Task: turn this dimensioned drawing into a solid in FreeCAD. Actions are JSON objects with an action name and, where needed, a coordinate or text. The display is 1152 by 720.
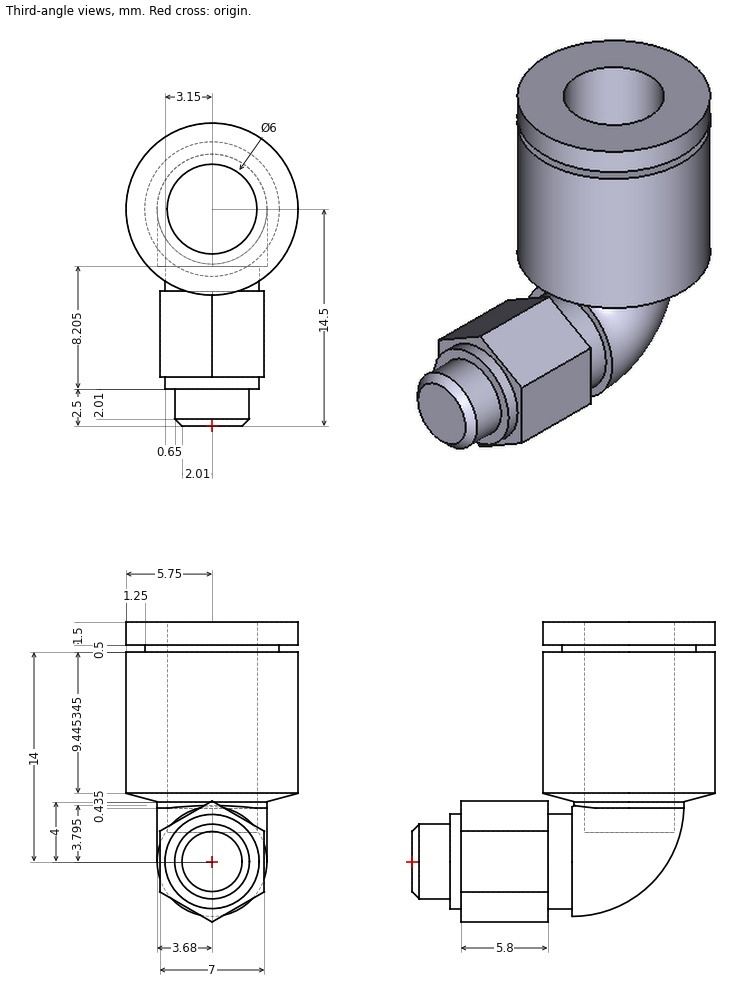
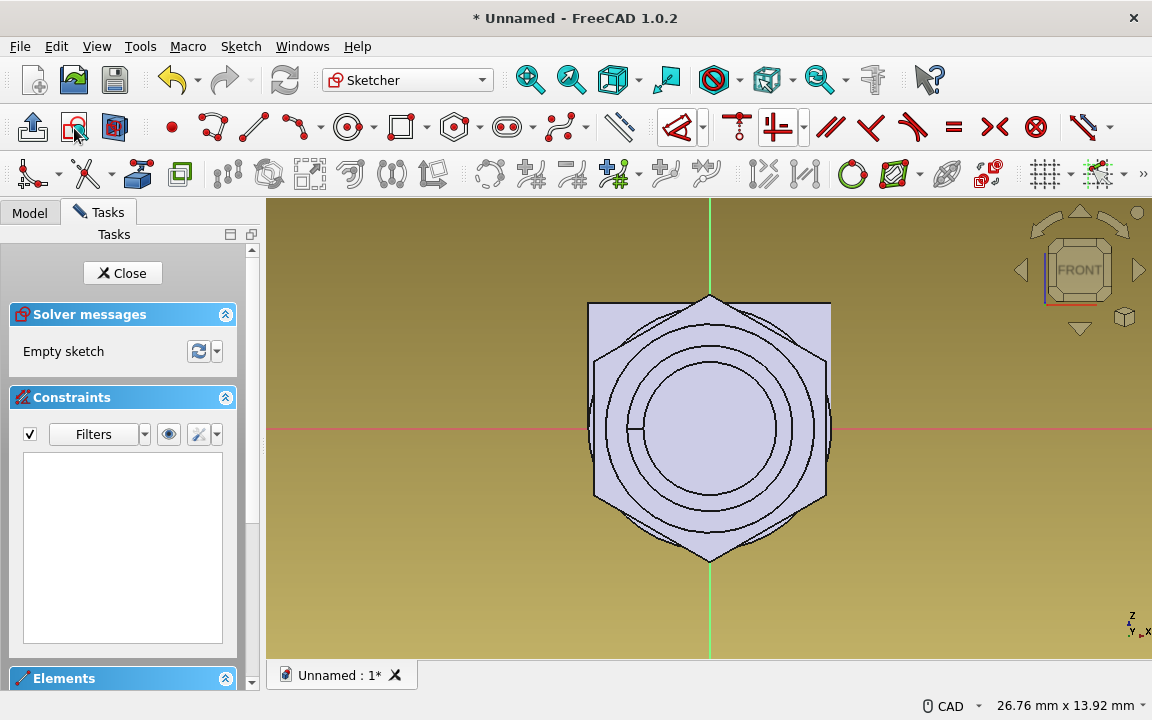
{"action": "left_click", "coordinate": [115, 128]}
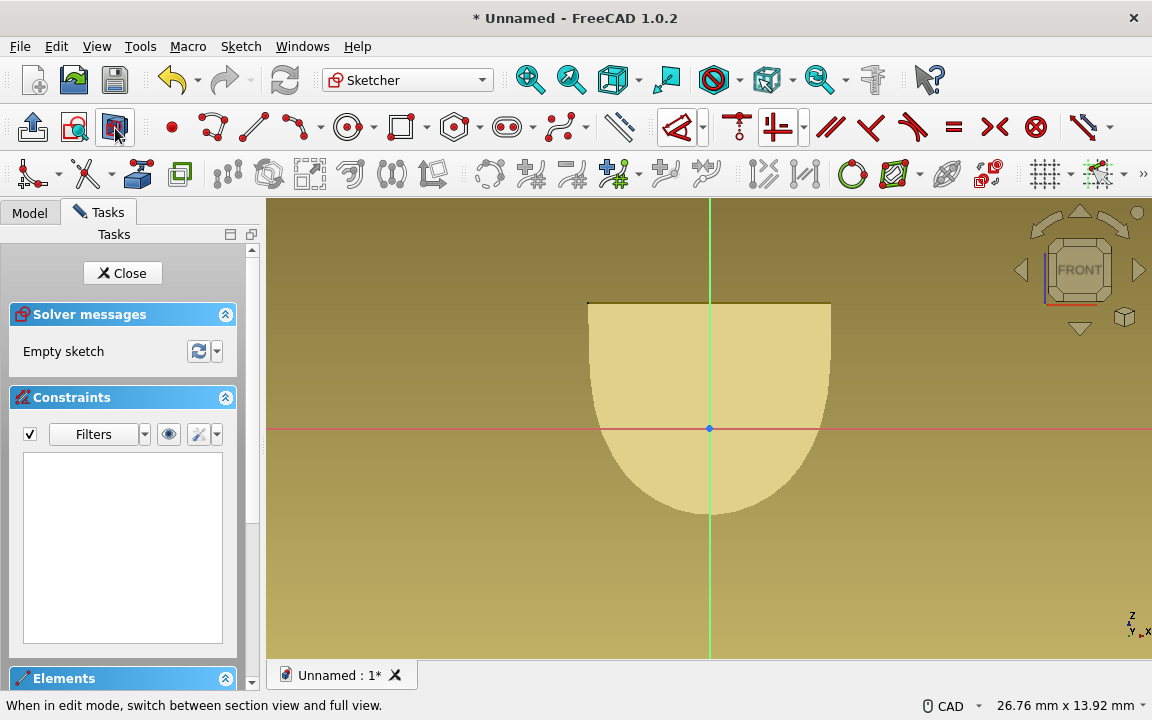
{"action": "scroll", "coordinate": [662, 631], "scroll_direction": "down", "scroll_amount": 4}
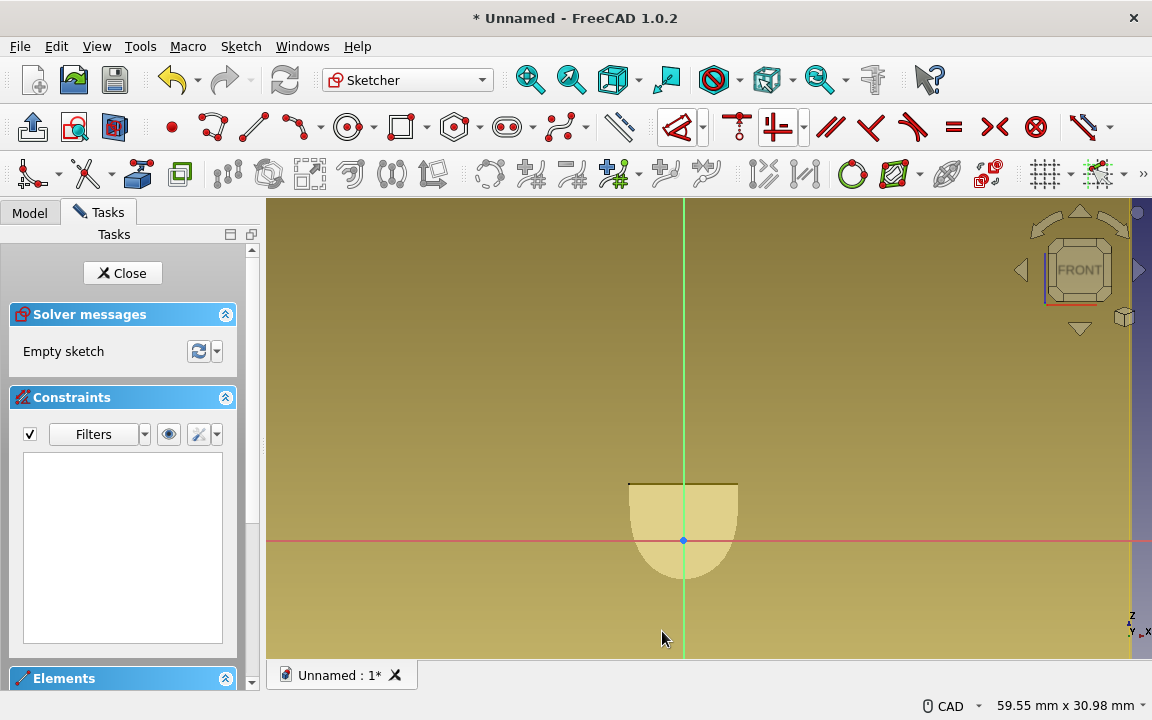
{"action": "left_click", "coordinate": [213, 128]}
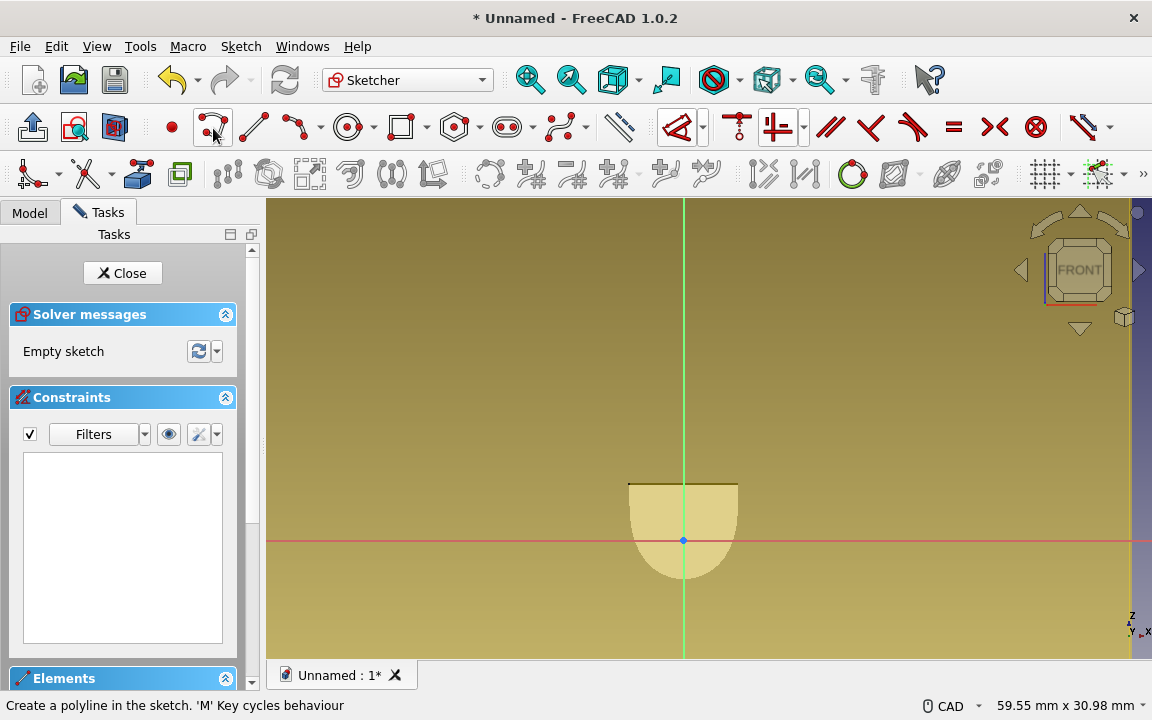
{"action": "left_click", "coordinate": [684, 487]}
{"action": "left_click", "coordinate": [629, 487]}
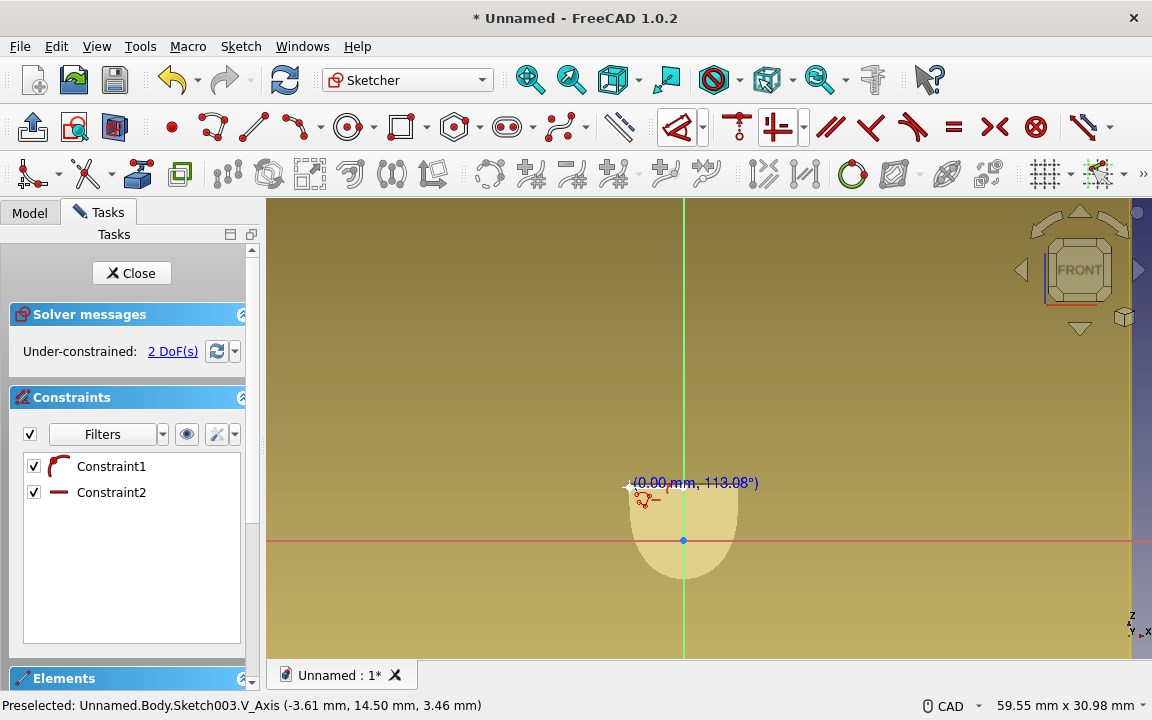
{"action": "scroll", "coordinate": [629, 481], "scroll_direction": "up", "scroll_amount": 5}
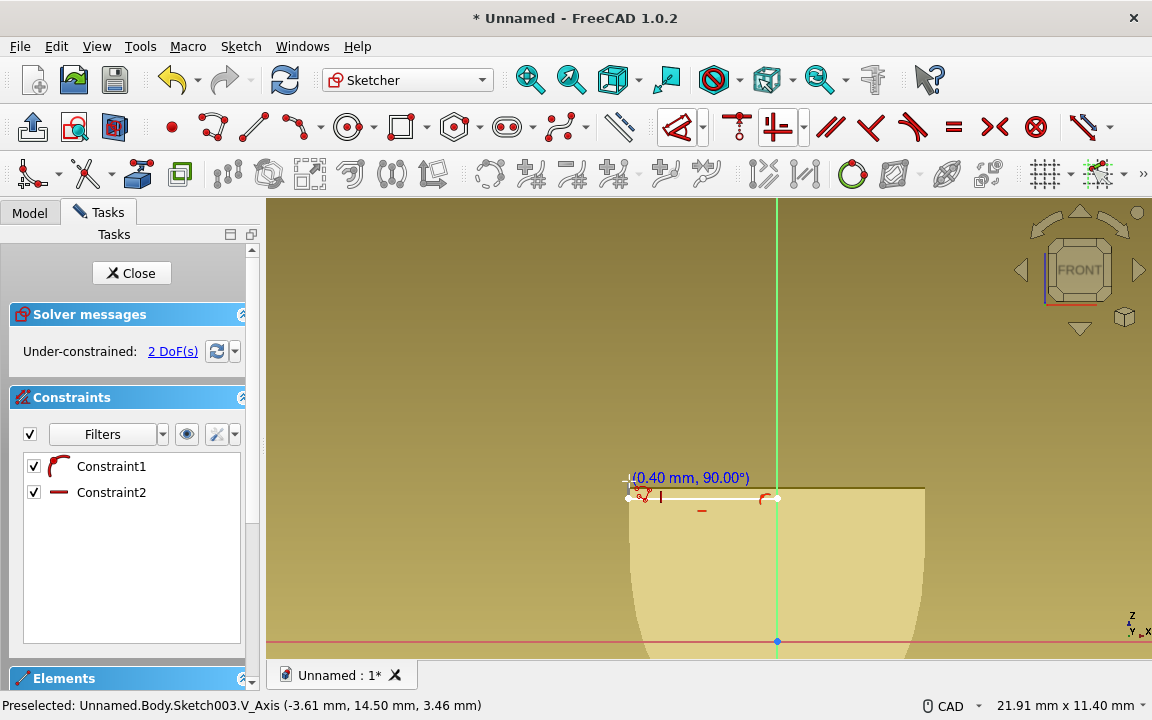
{"action": "left_click", "coordinate": [628, 480]}
{"action": "left_click", "coordinate": [545, 458]}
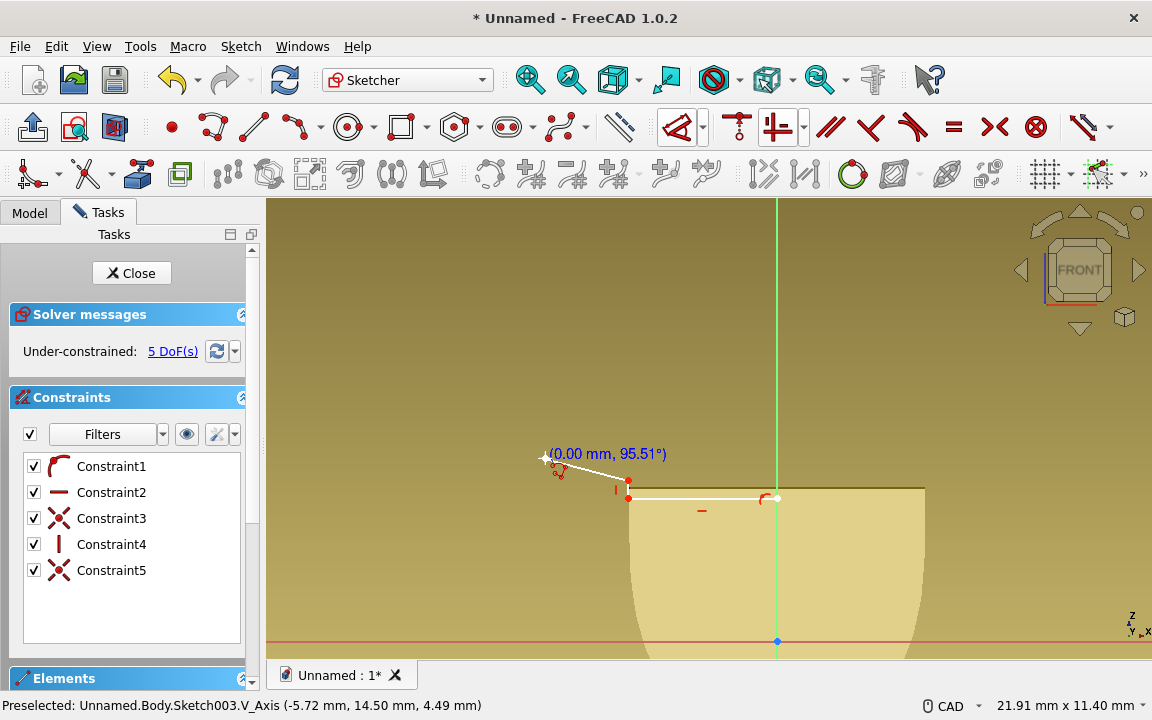
{"action": "scroll", "coordinate": [624, 518], "scroll_direction": "down", "scroll_amount": 4}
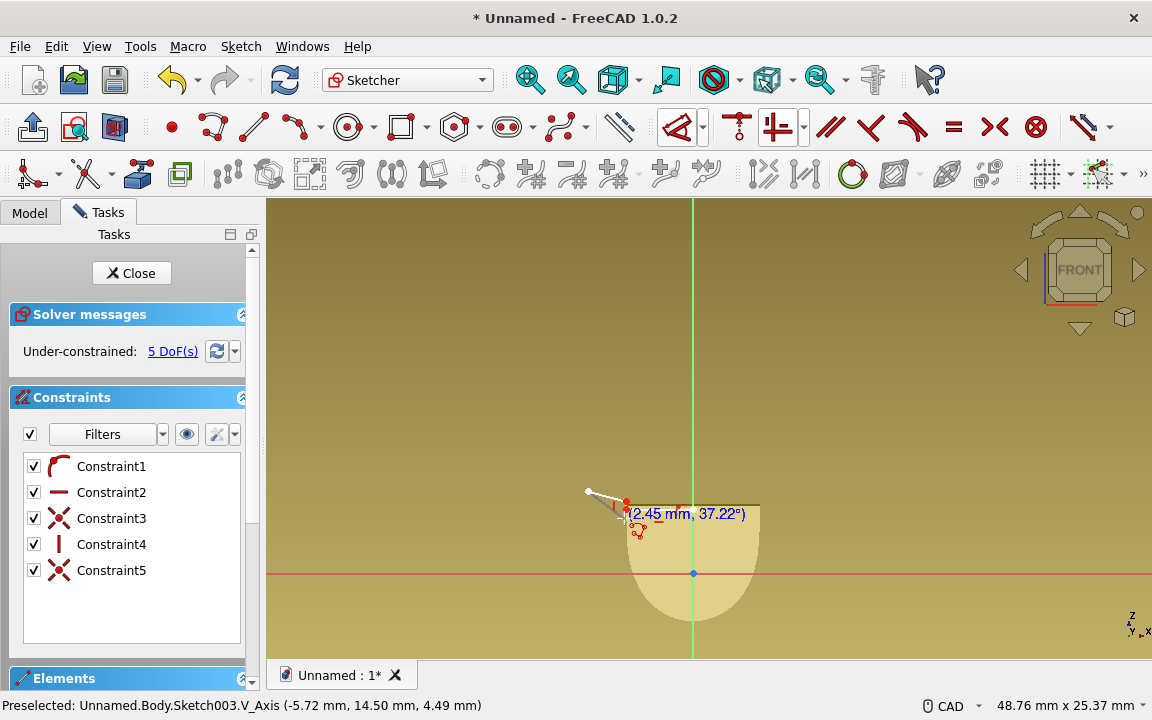
{"action": "left_click", "coordinate": [589, 320]}
{"action": "left_click", "coordinate": [611, 320]}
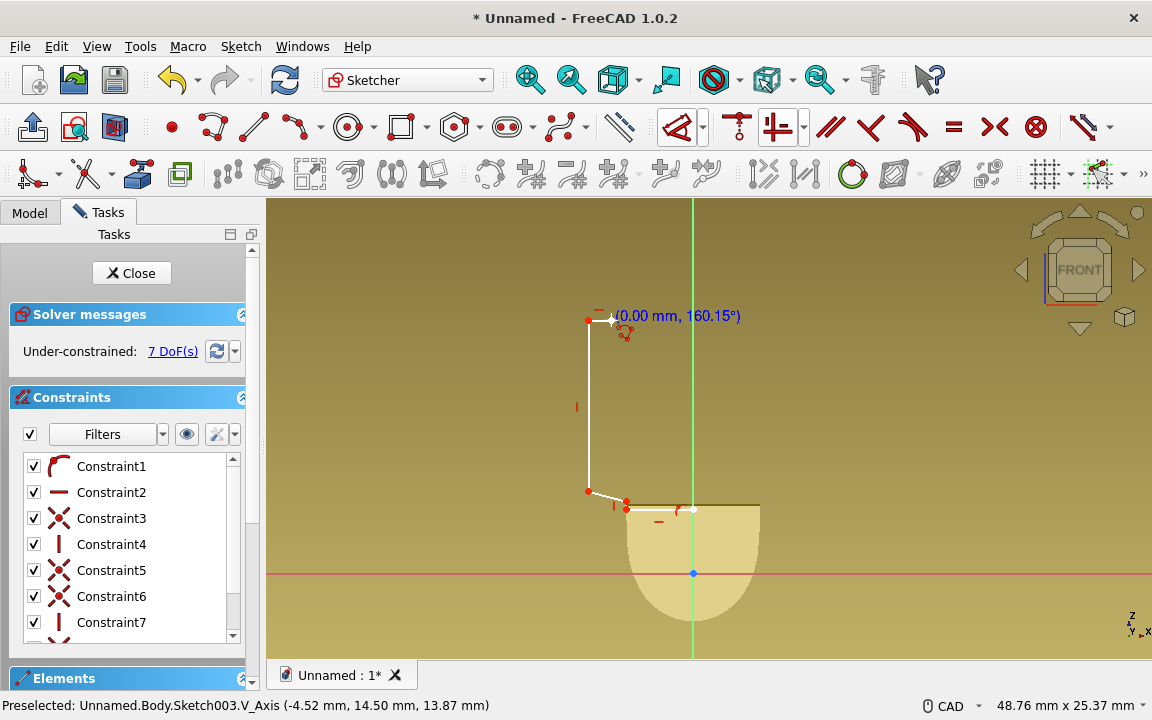
{"action": "scroll", "coordinate": [611, 310], "scroll_direction": "up", "scroll_amount": 3}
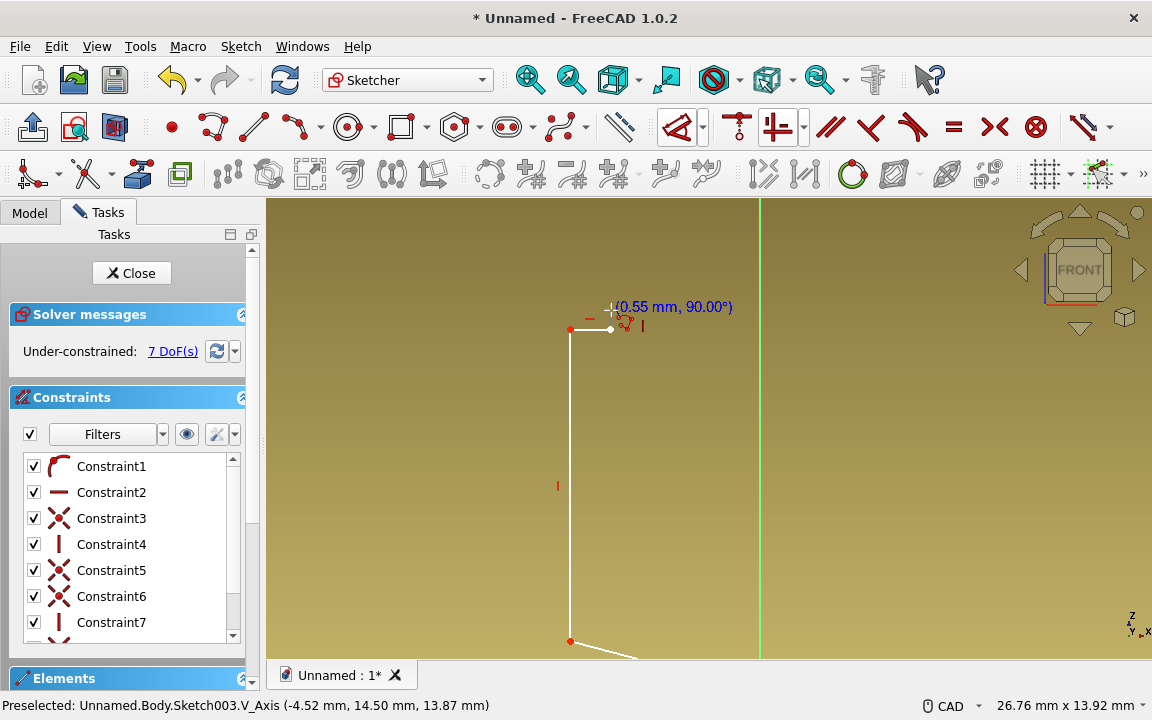
{"action": "left_click", "coordinate": [611, 311]}
{"action": "left_click", "coordinate": [570, 311]}
{"action": "left_click", "coordinate": [570, 261]}
{"action": "left_click", "coordinate": [751, 261]}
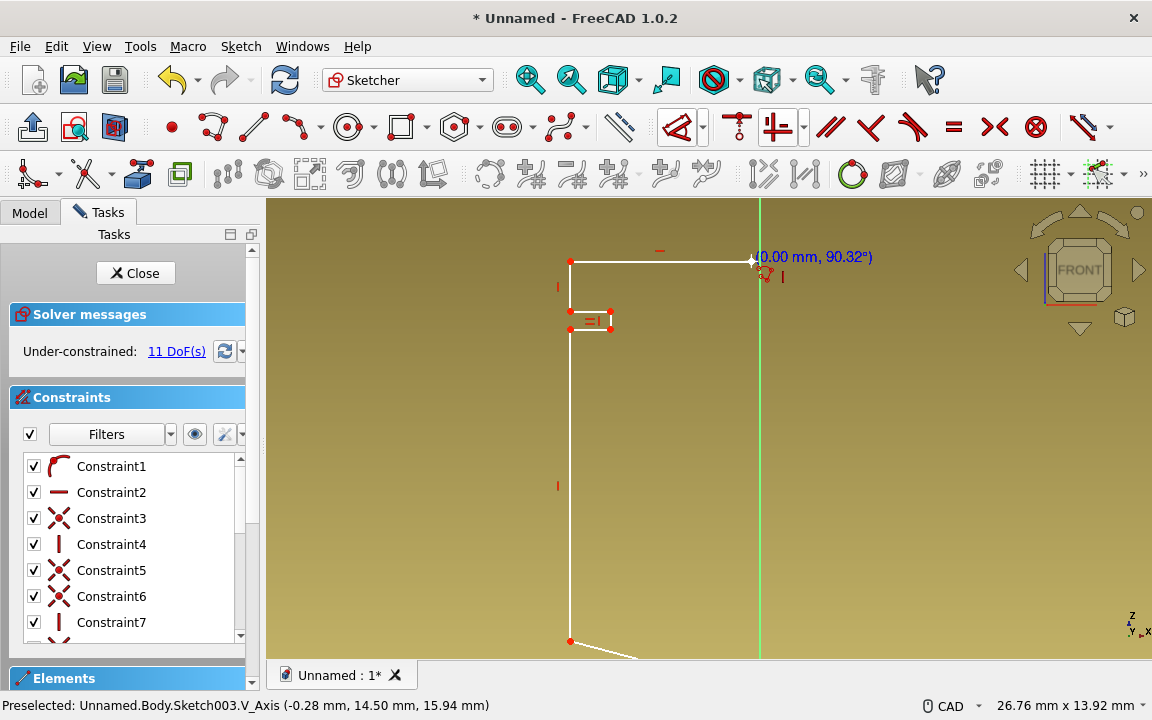
{"action": "scroll", "coordinate": [611, 310], "scroll_direction": "down", "scroll_amount": 3}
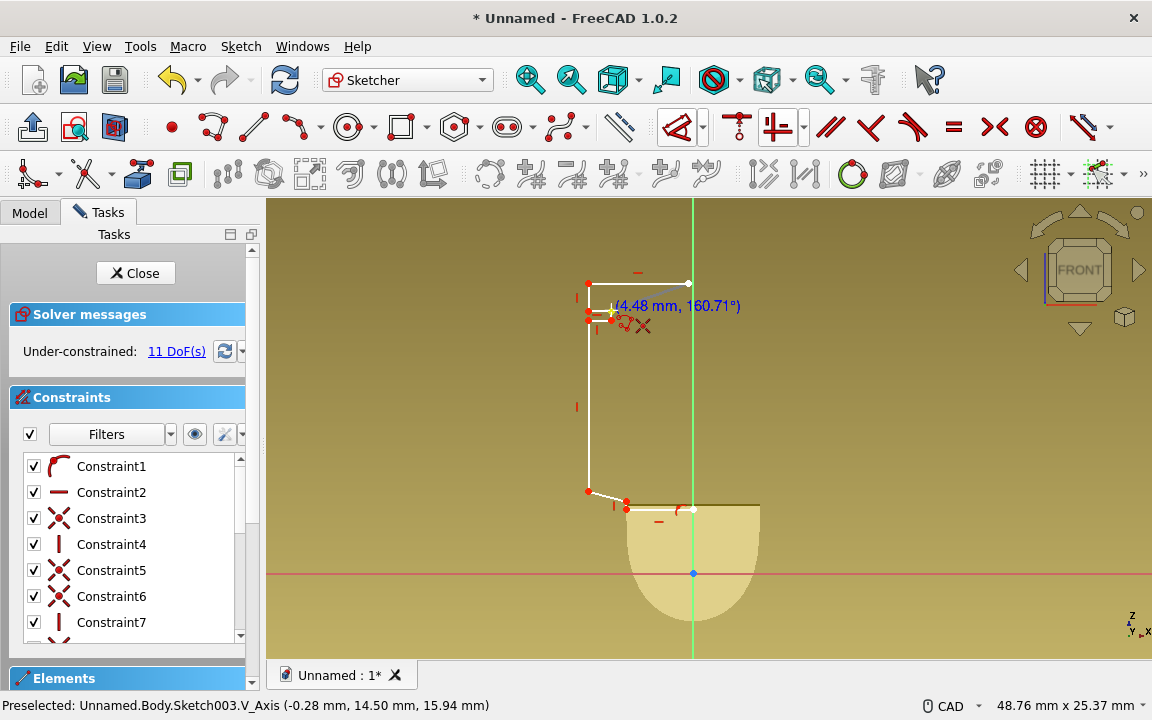
{"action": "left_click", "coordinate": [693, 510]}
{"action": "key", "text": "Escape"}
{"action": "key", "text": "Escape"}